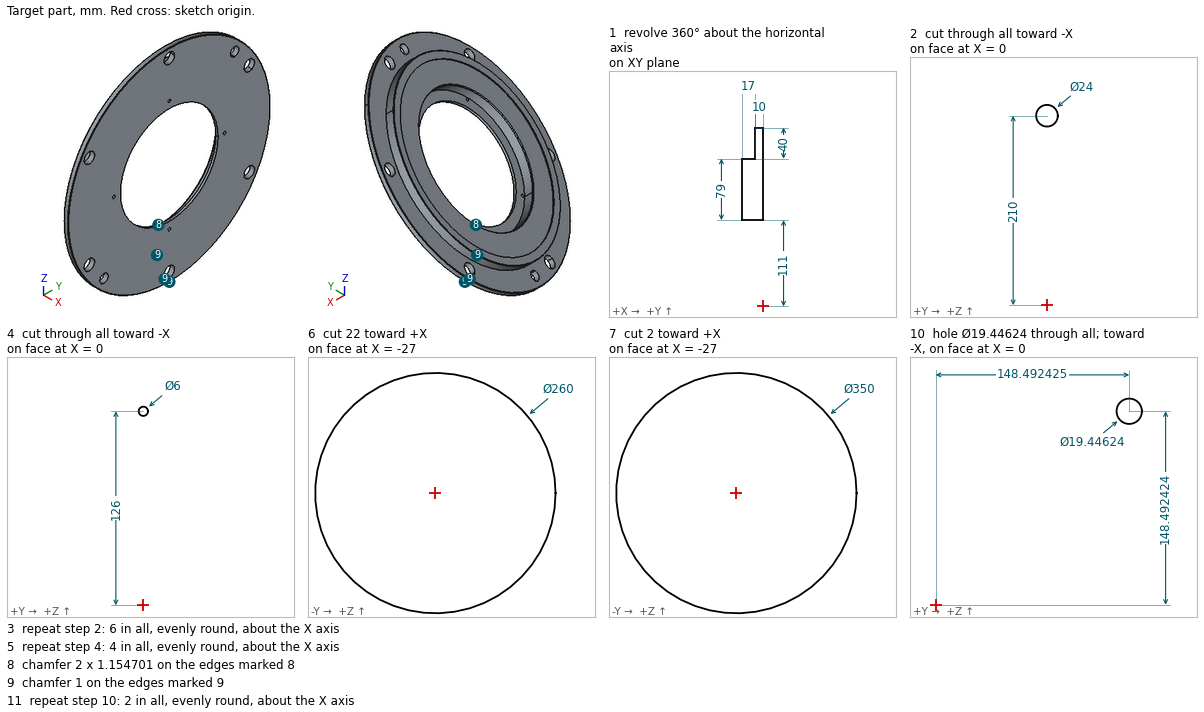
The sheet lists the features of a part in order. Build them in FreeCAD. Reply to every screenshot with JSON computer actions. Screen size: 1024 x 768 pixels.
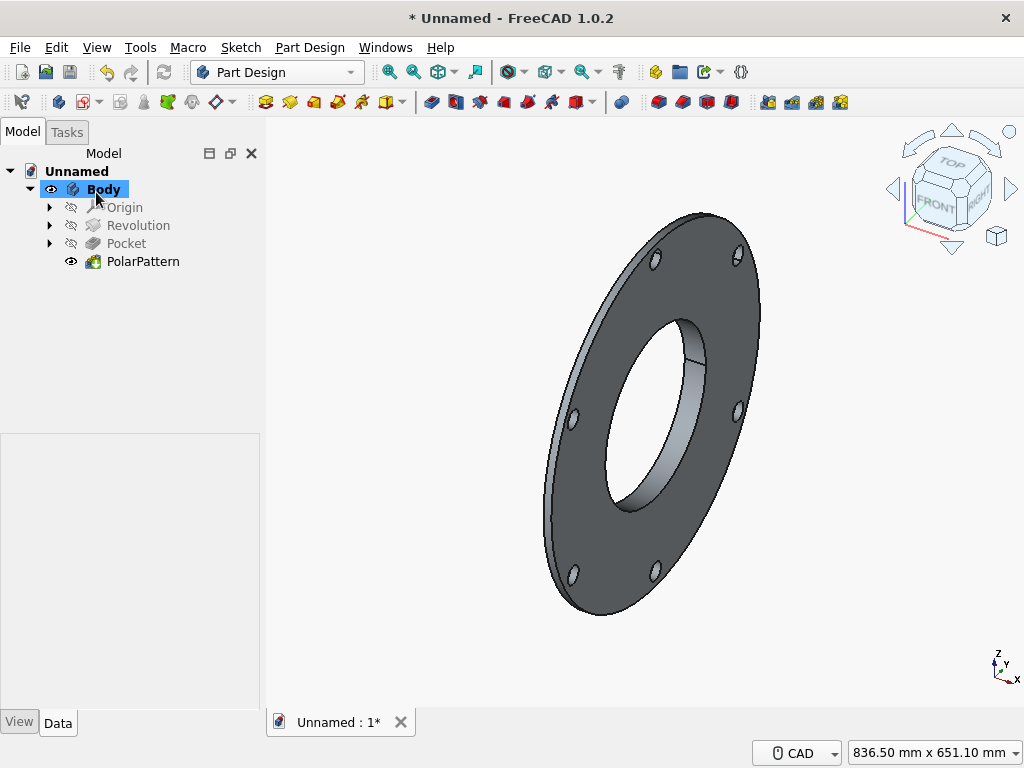
{"action": "left_click", "coordinate": [596, 571]}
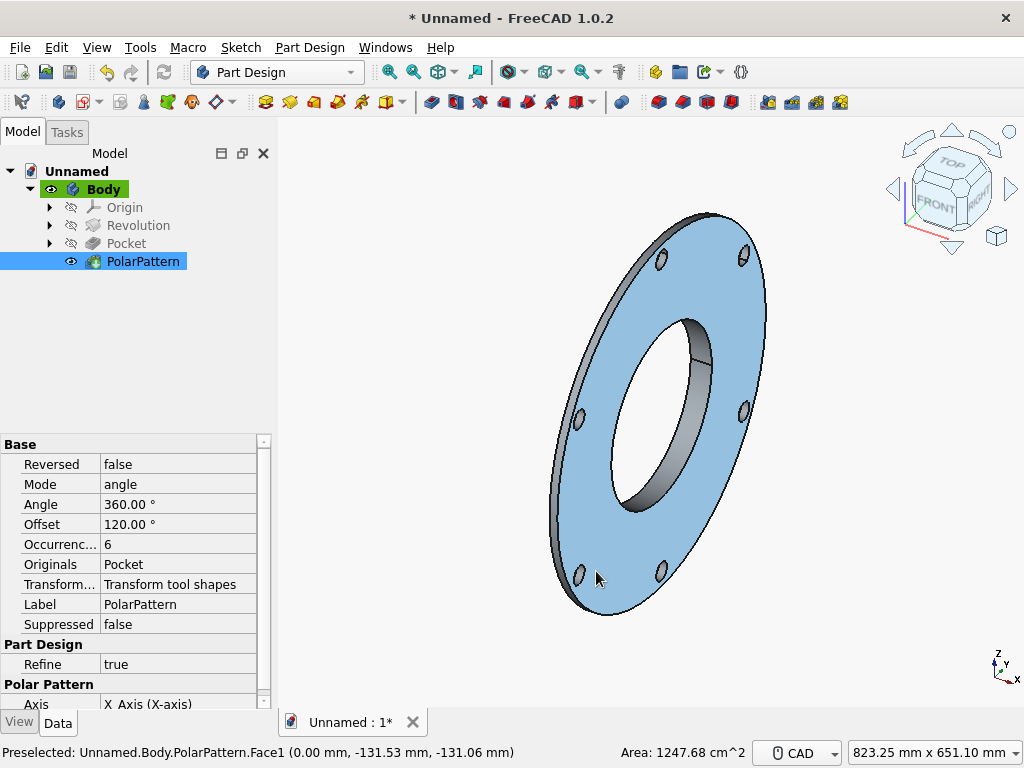
{"action": "left_click", "coordinate": [84, 102]}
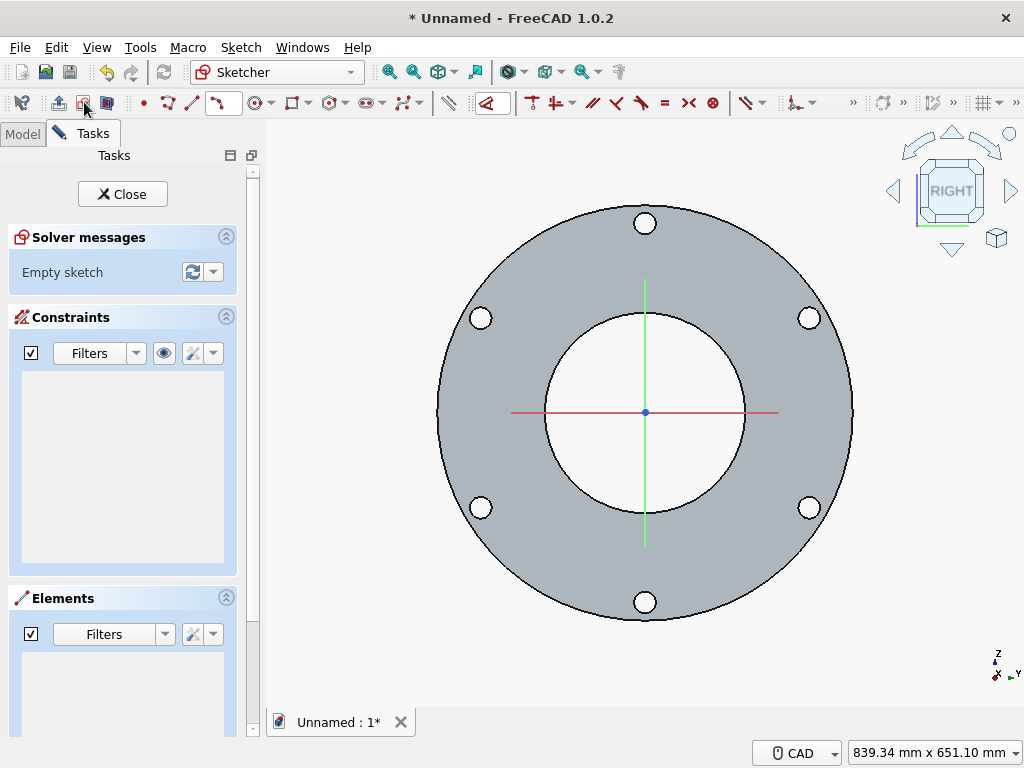
{"action": "scroll", "coordinate": [649, 293], "scroll_direction": "up", "scroll_amount": 15}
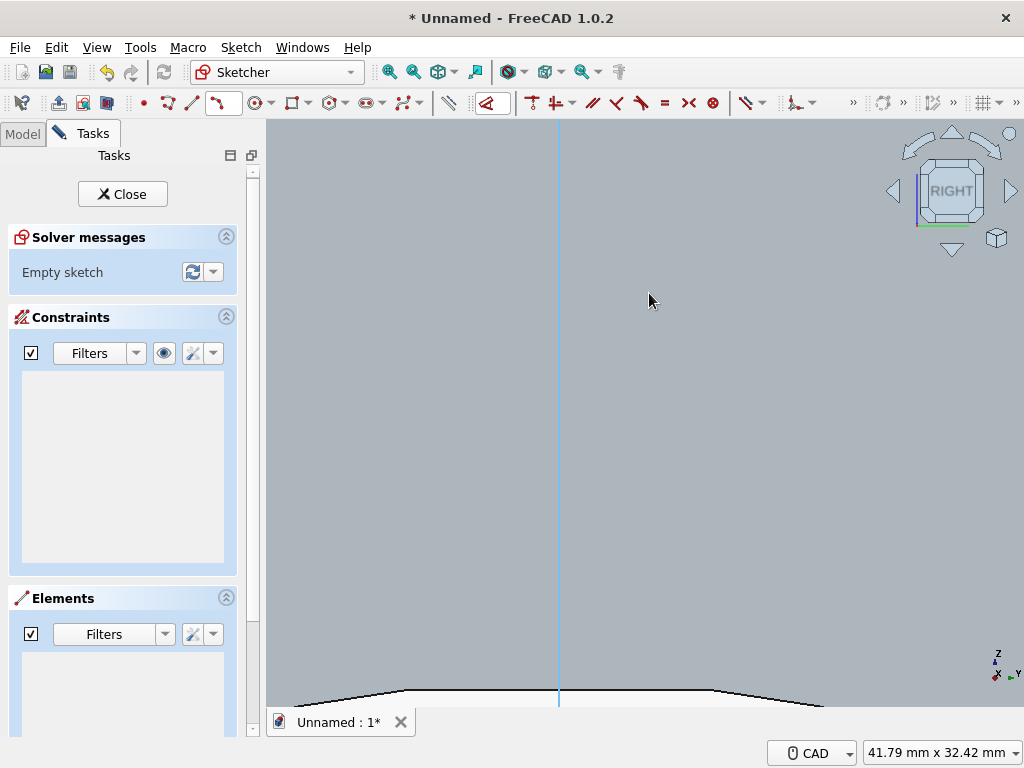
{"action": "scroll", "coordinate": [551, 412], "scroll_direction": "up", "scroll_amount": 6}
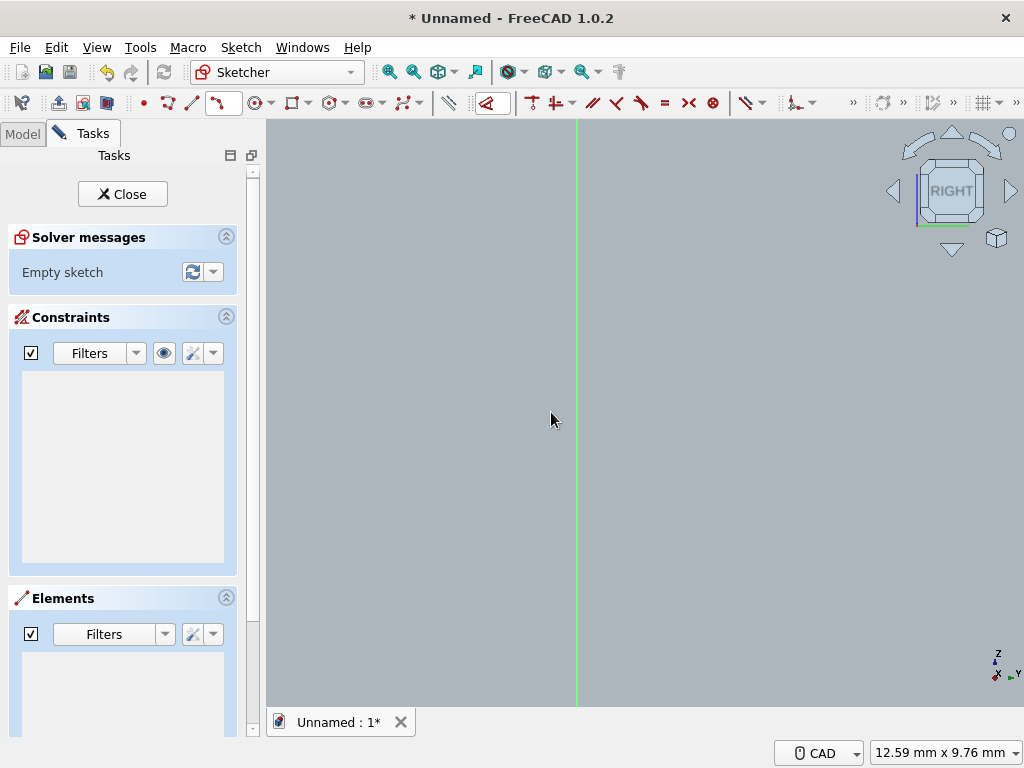
{"action": "left_click", "coordinate": [256, 104]}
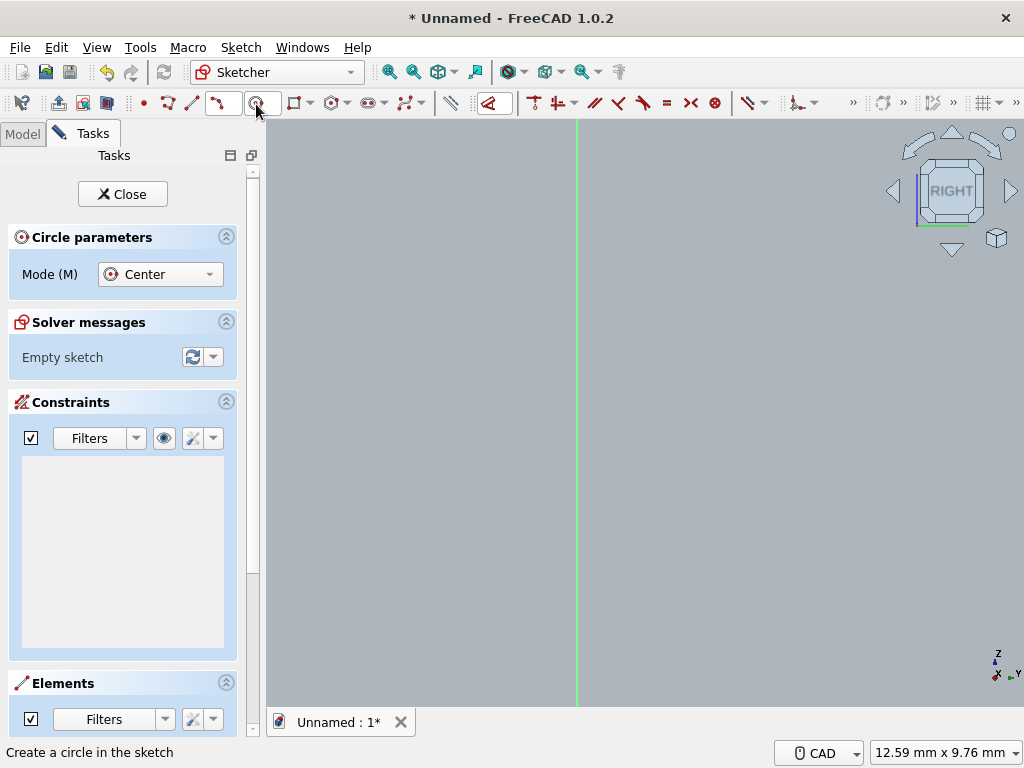
{"action": "left_click", "coordinate": [577, 411]}
{"action": "mouse_move", "coordinate": [704, 283]}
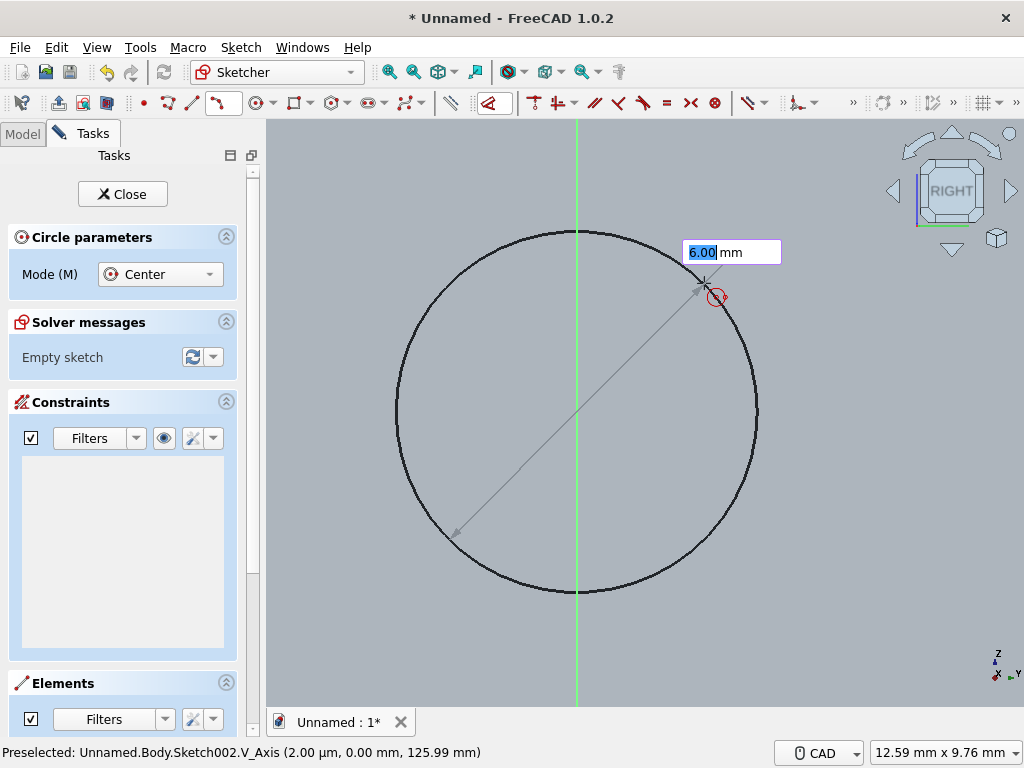
{"action": "type", "text": "6"}
{"action": "key", "text": "Return"}
{"action": "key", "text": "Escape"}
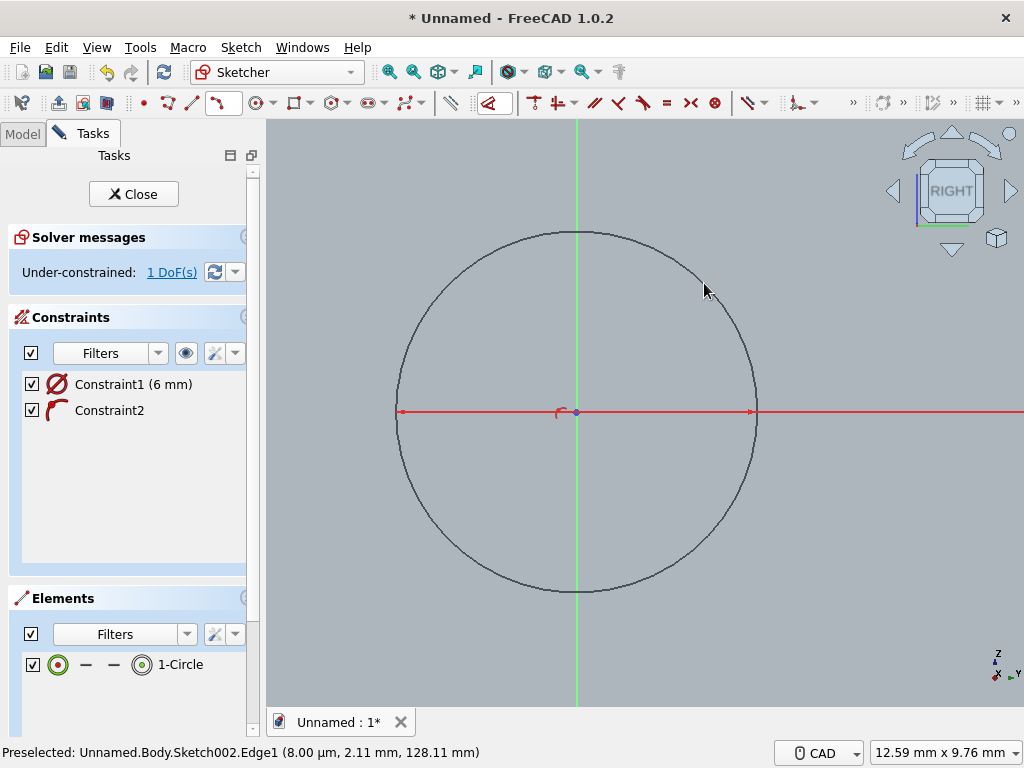
{"action": "key", "text": "d"}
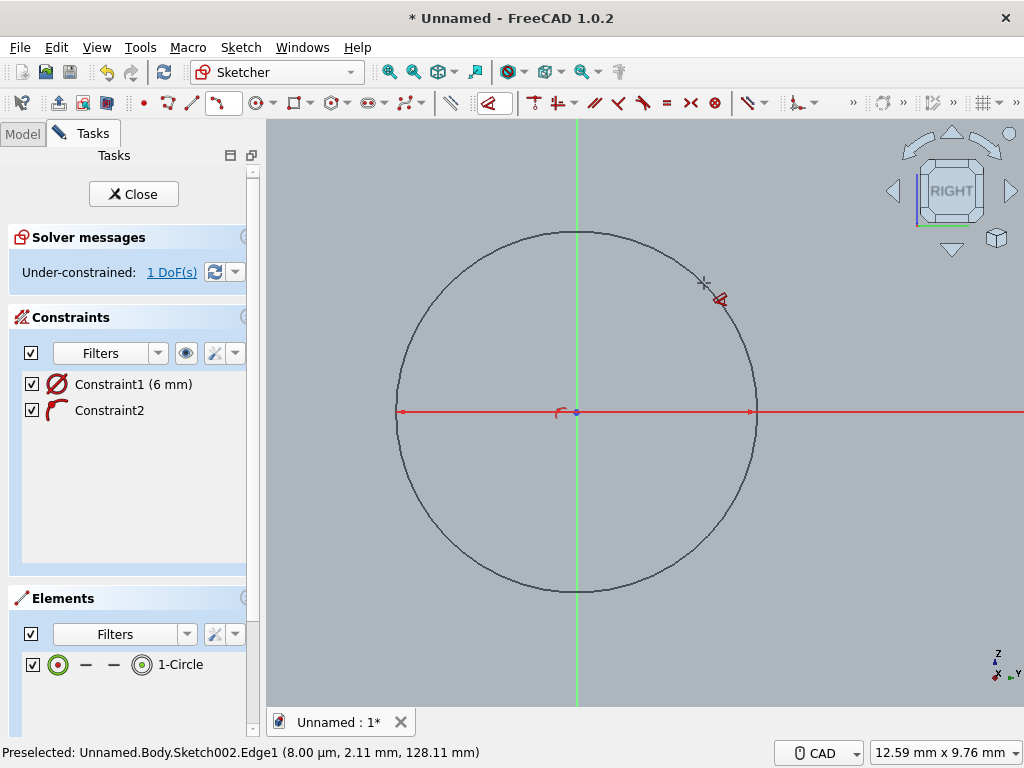
{"action": "left_click", "coordinate": [577, 412]}
{"action": "left_click", "coordinate": [611, 546]}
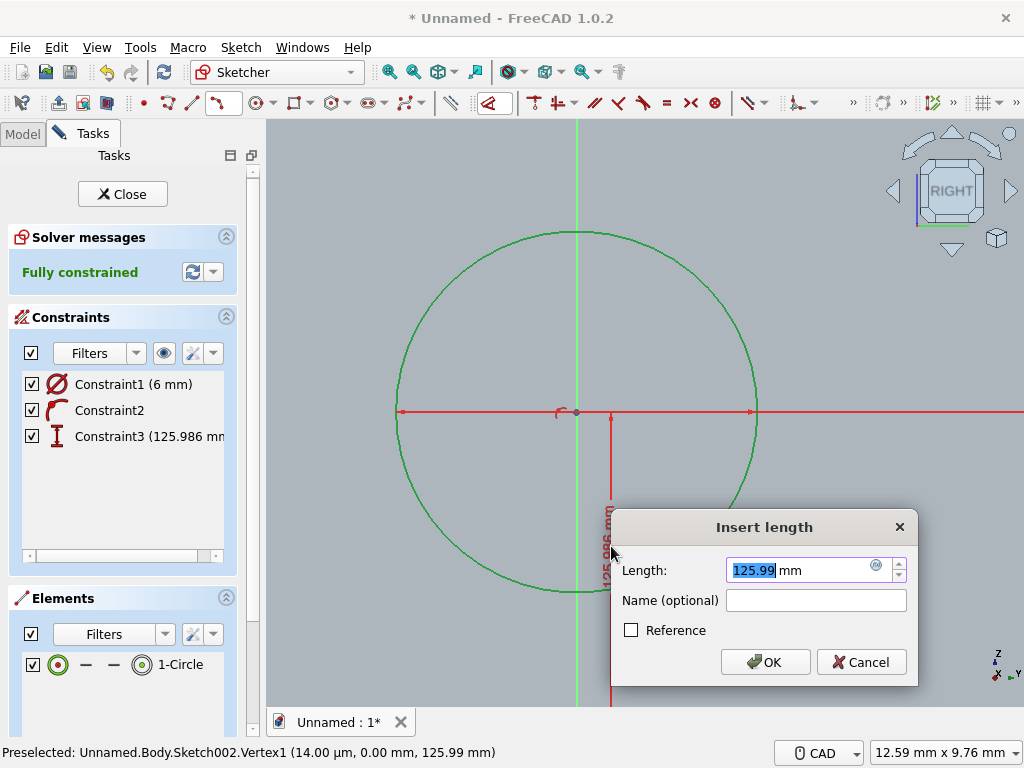
{"action": "type", "text": "126"}
{"action": "key", "text": "Return"}
{"action": "key", "text": "Escape"}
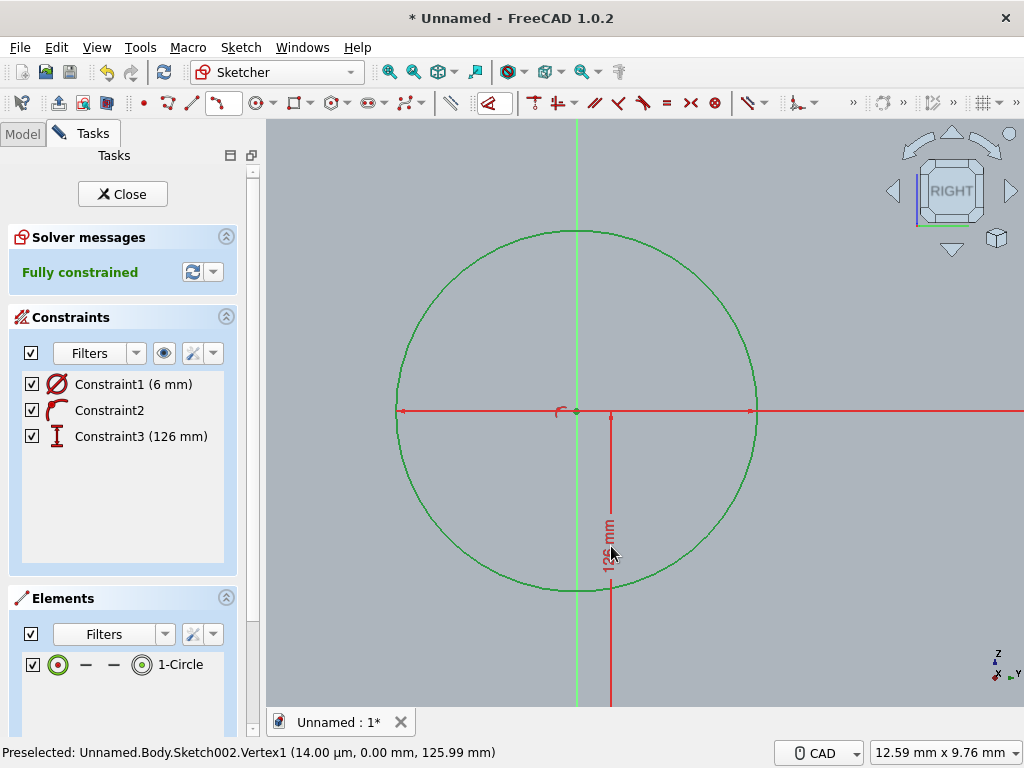
{"action": "left_click", "coordinate": [123, 194]}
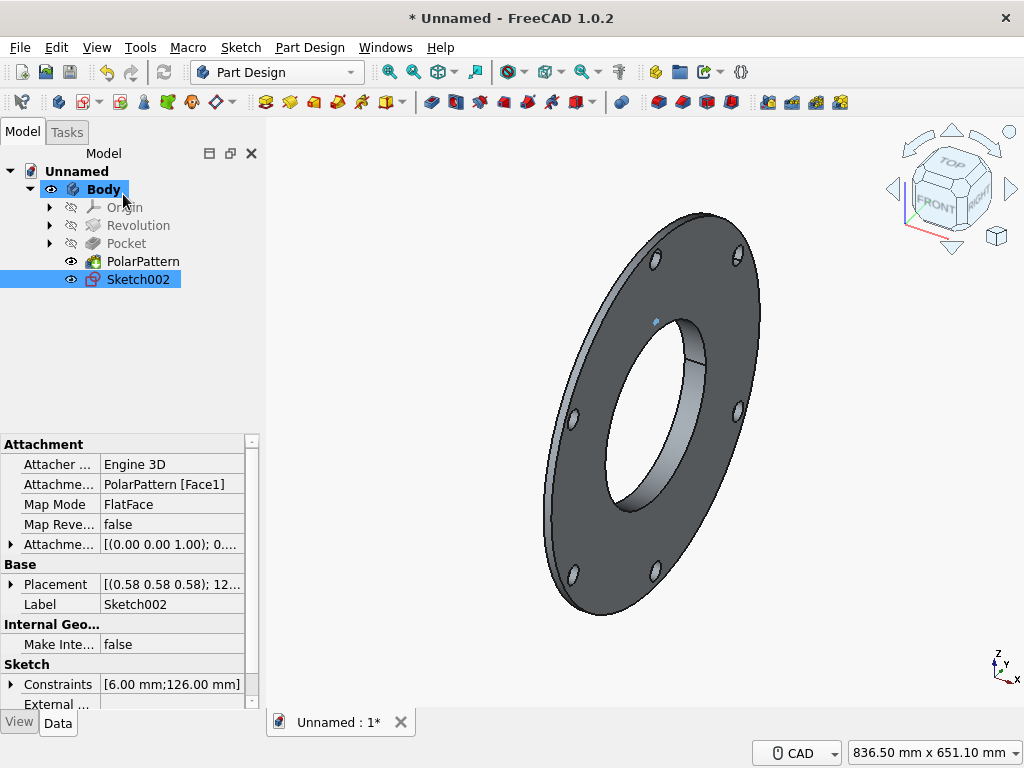
{"action": "left_click", "coordinate": [432, 102]}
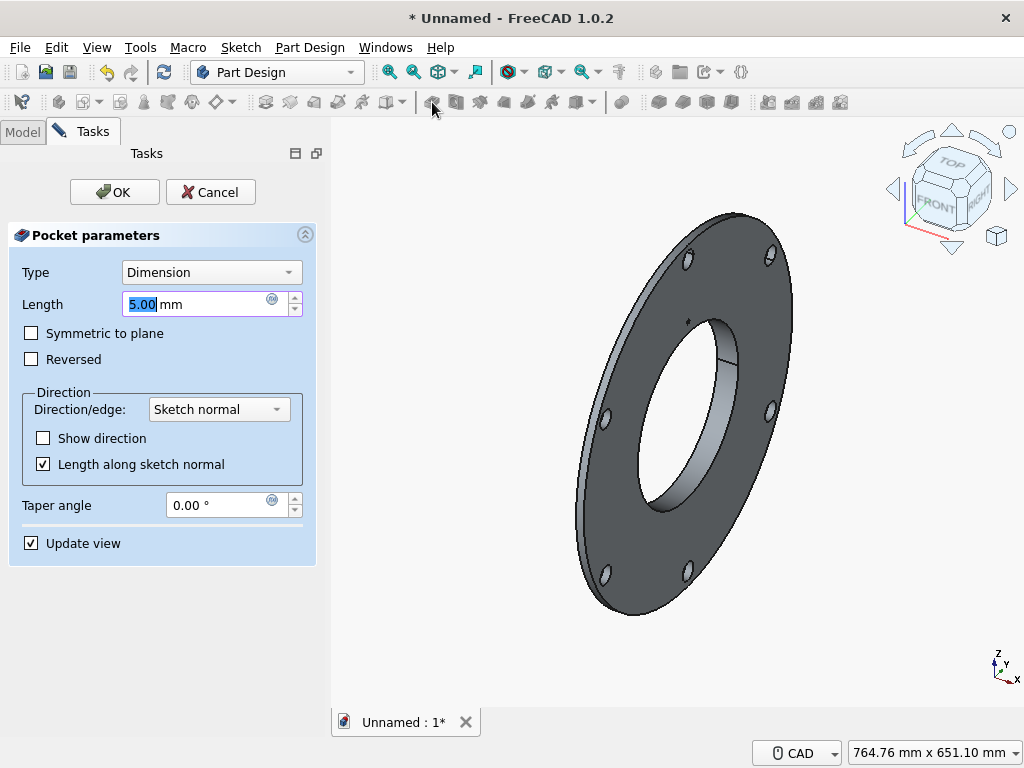
{"action": "left_click", "coordinate": [212, 272]}